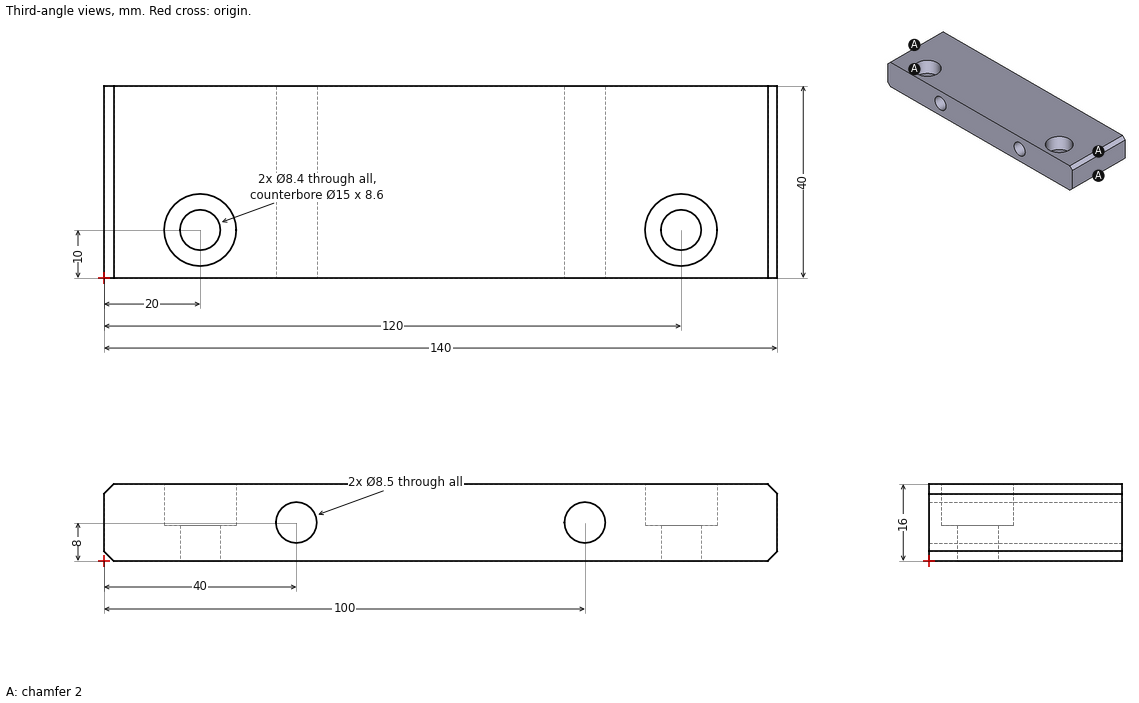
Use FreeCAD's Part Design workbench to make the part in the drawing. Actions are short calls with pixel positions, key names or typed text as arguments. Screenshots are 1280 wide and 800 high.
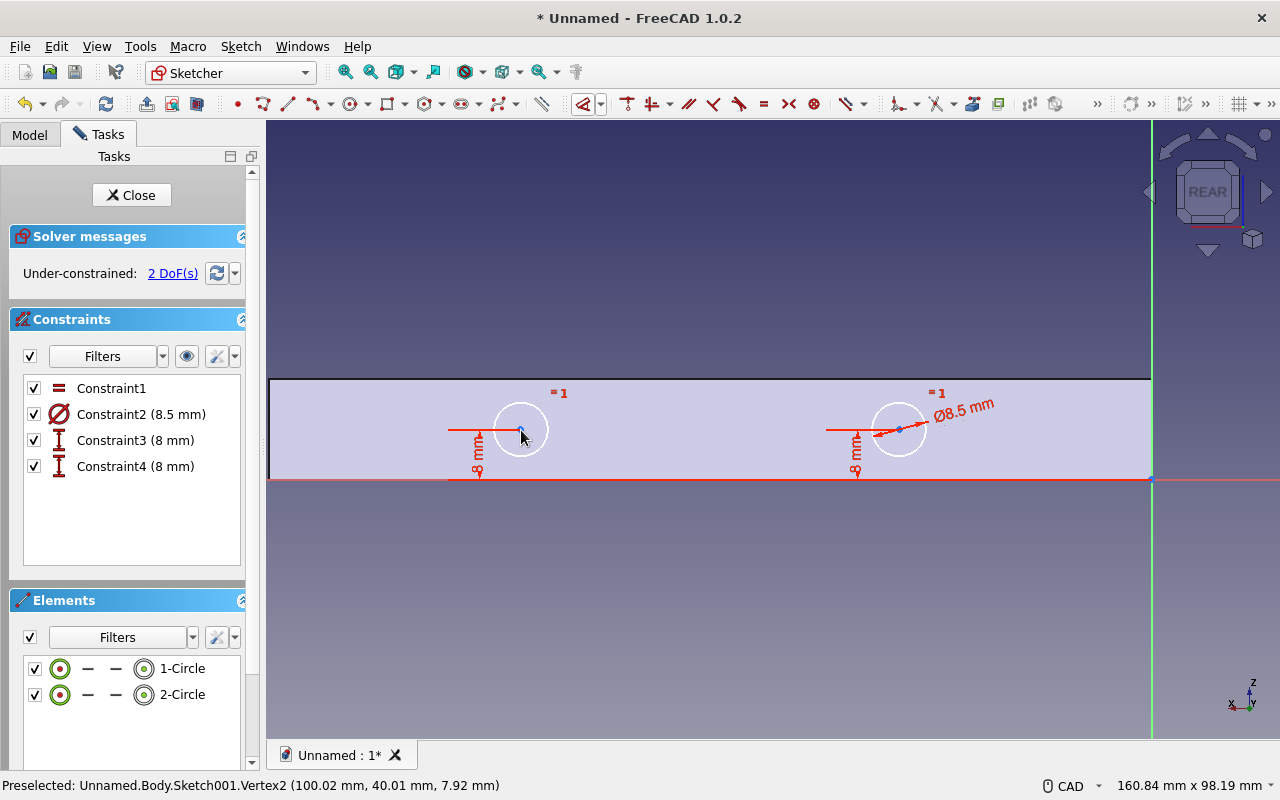
click(899, 429)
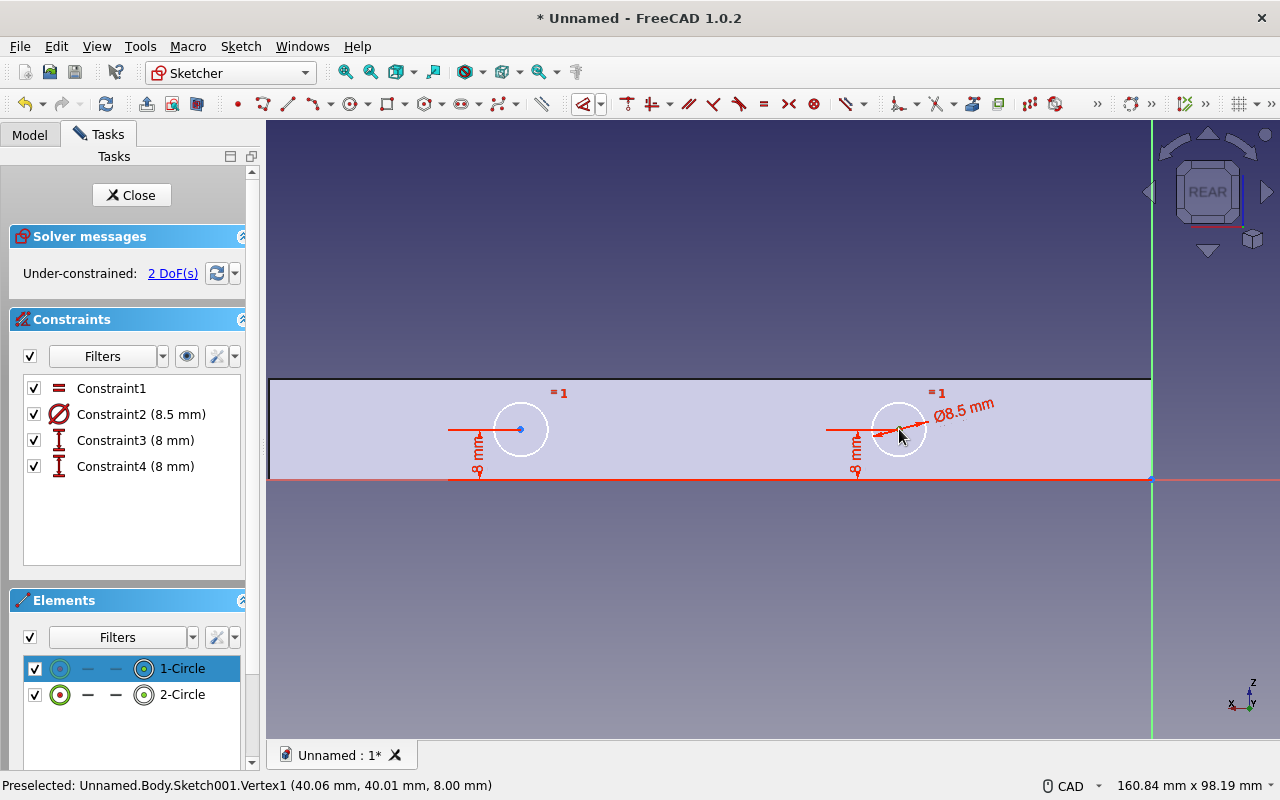
key(l)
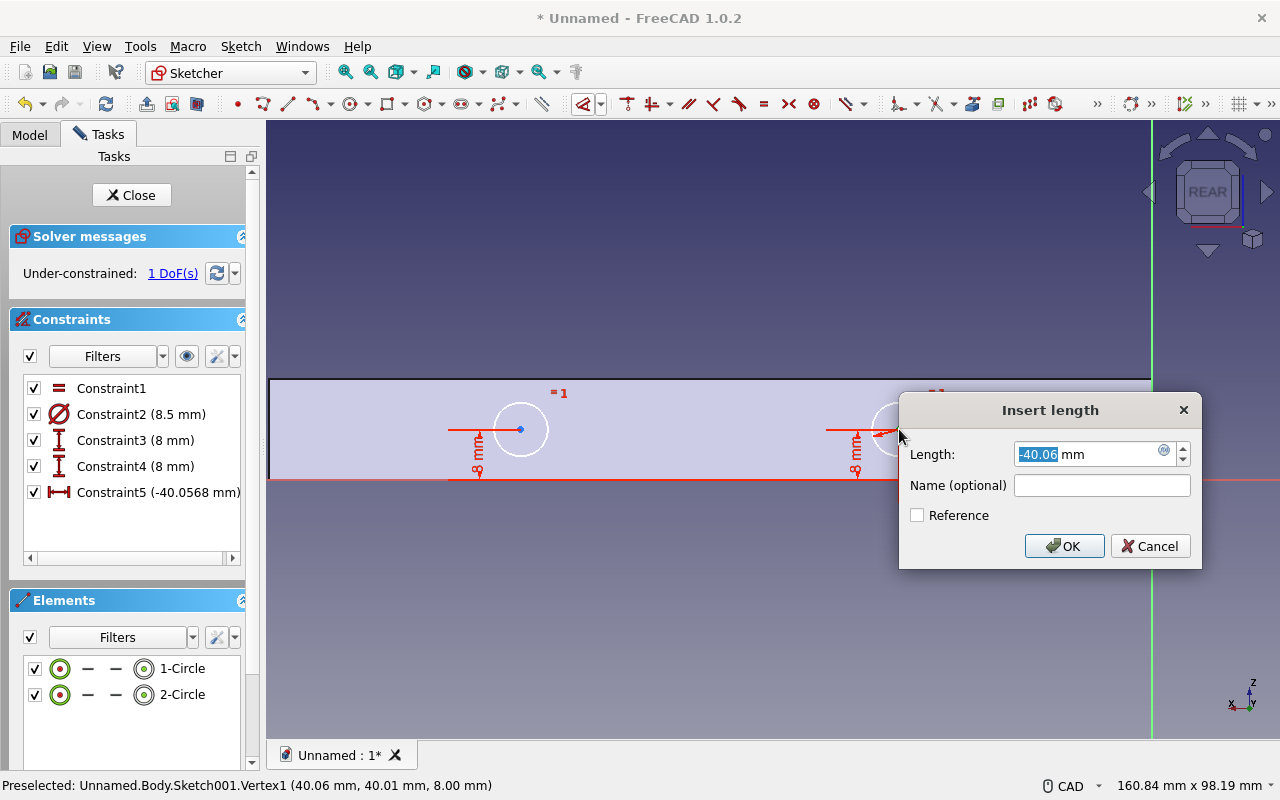
text(-40)
key(Return)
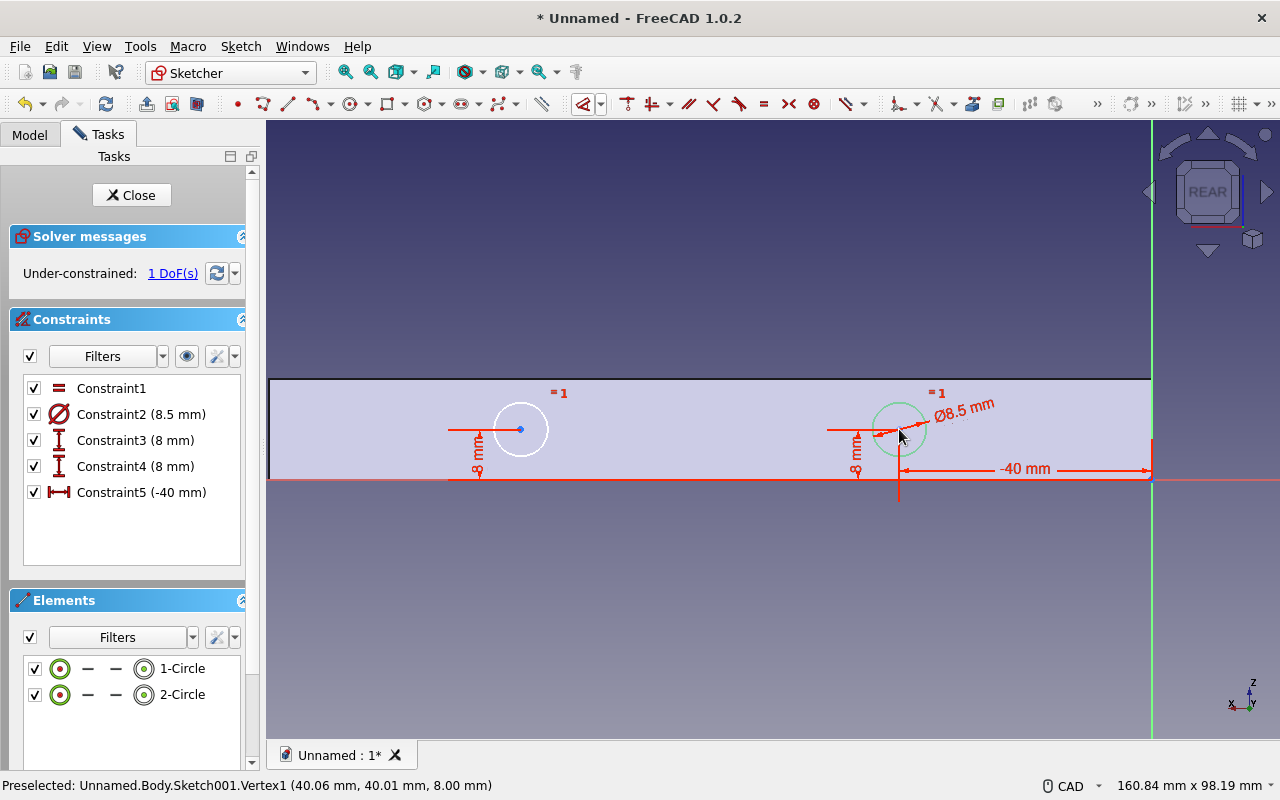
click(521, 429)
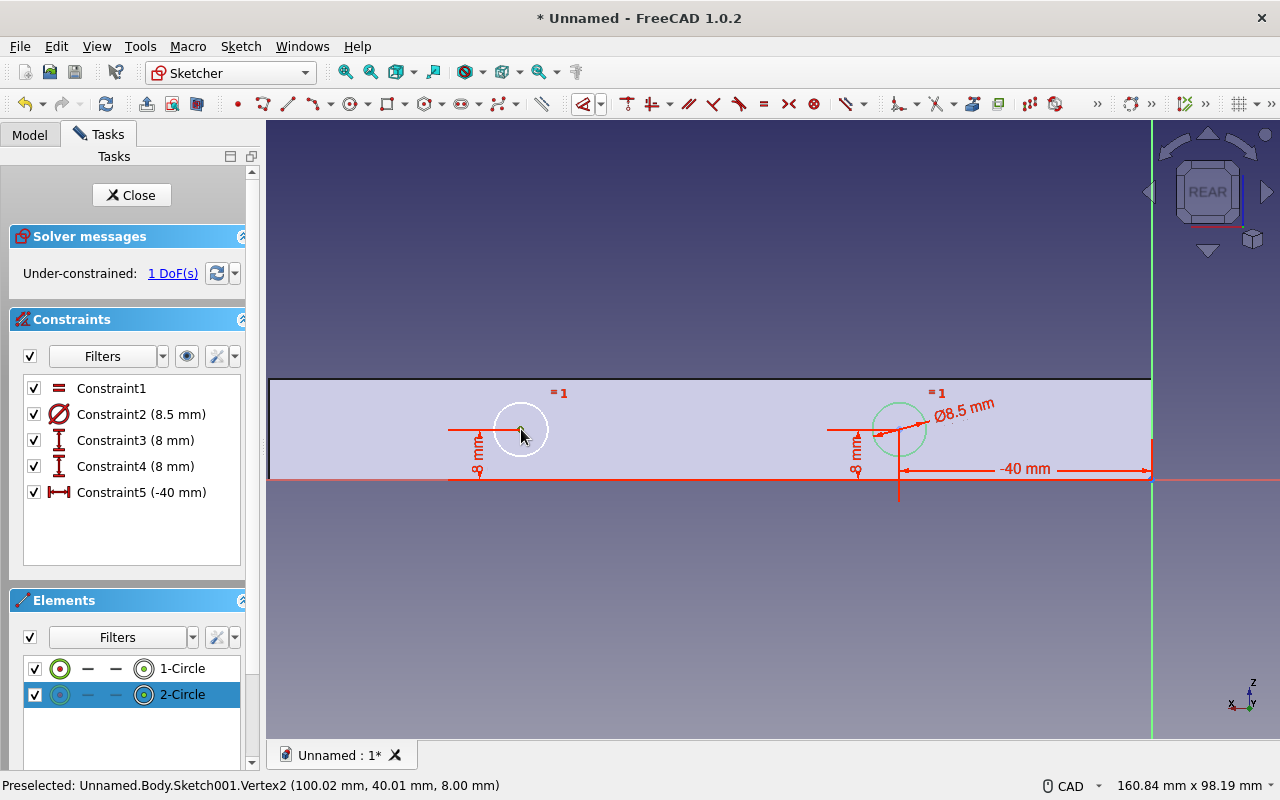
key(l)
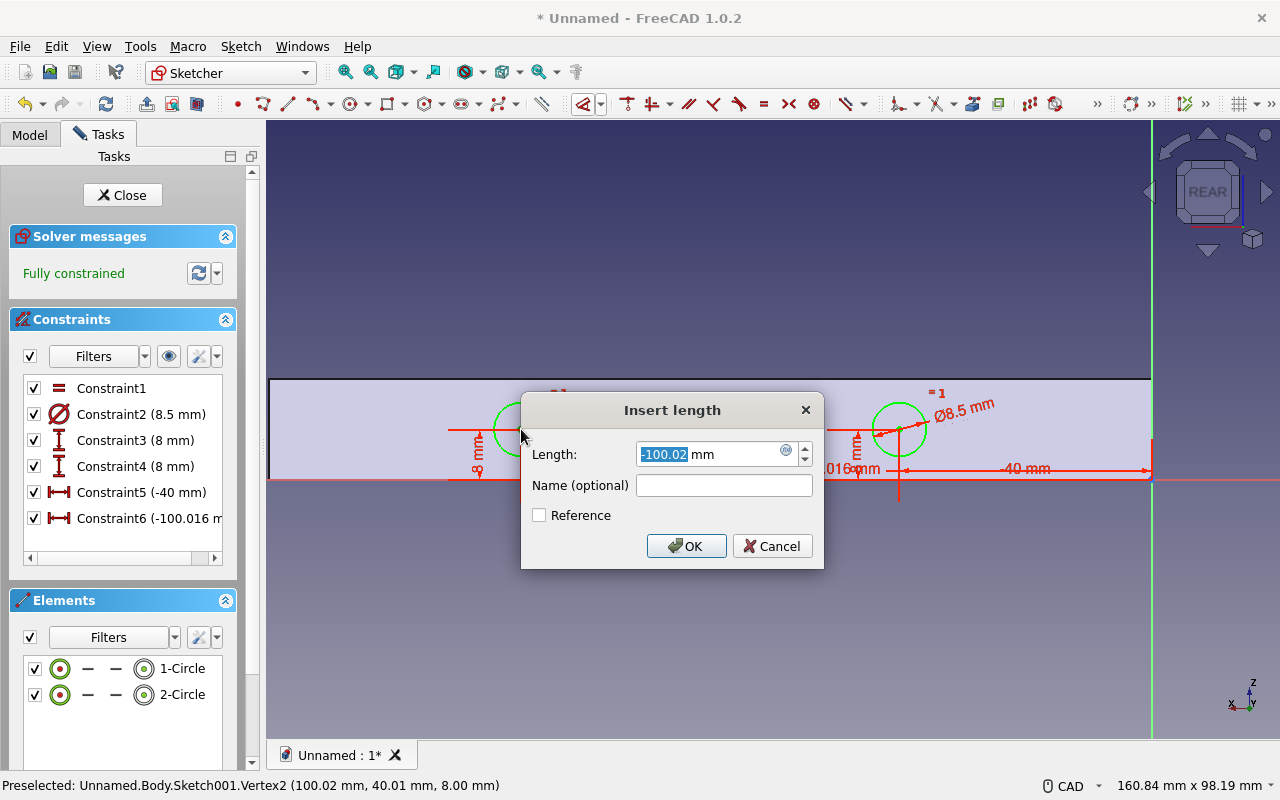
text(-100)
key(Return)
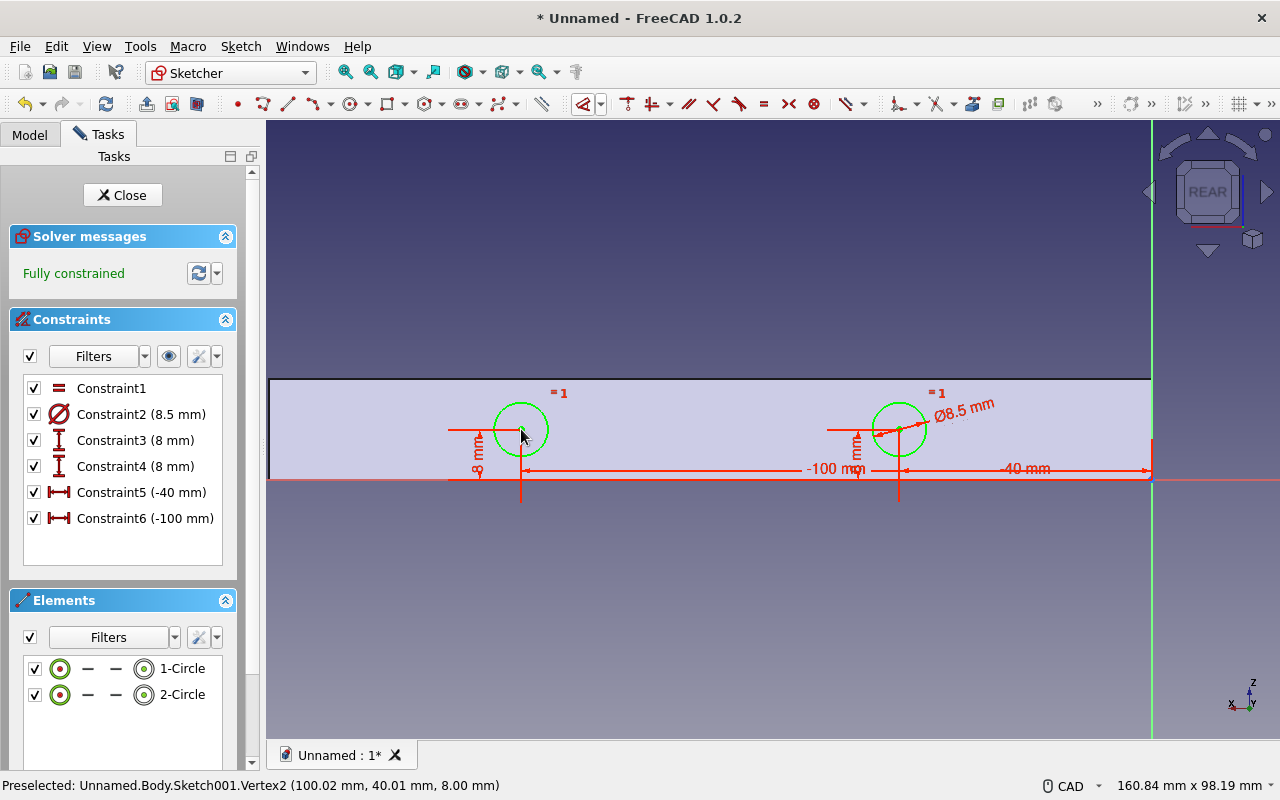
click(123, 195)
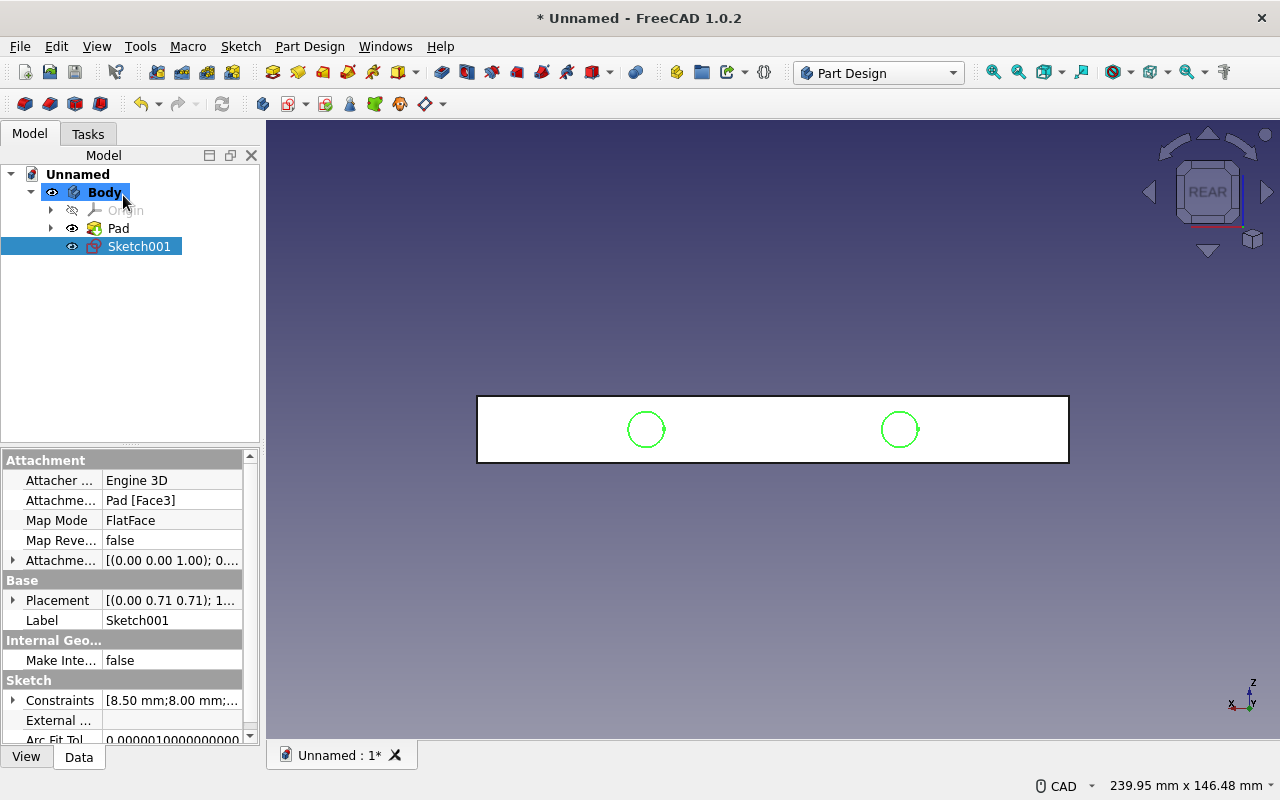
click(467, 72)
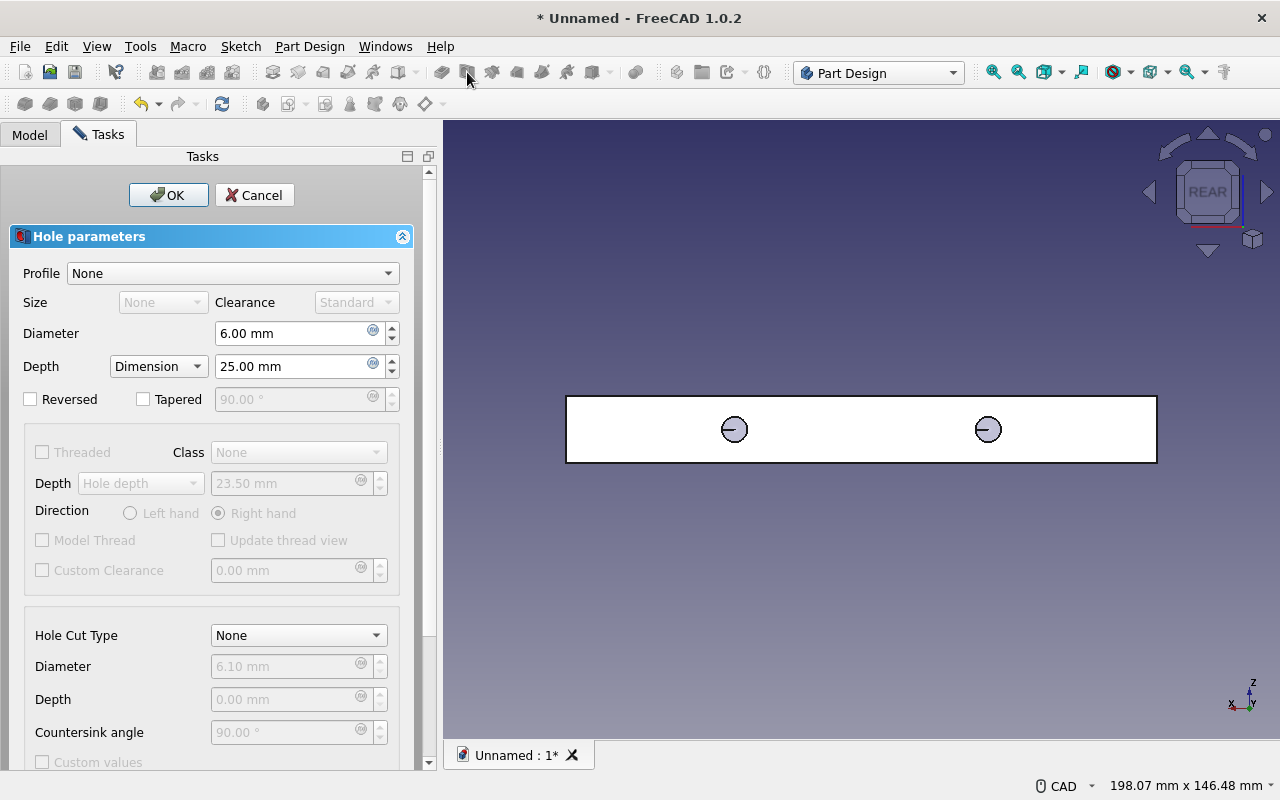
triple_click(300, 334)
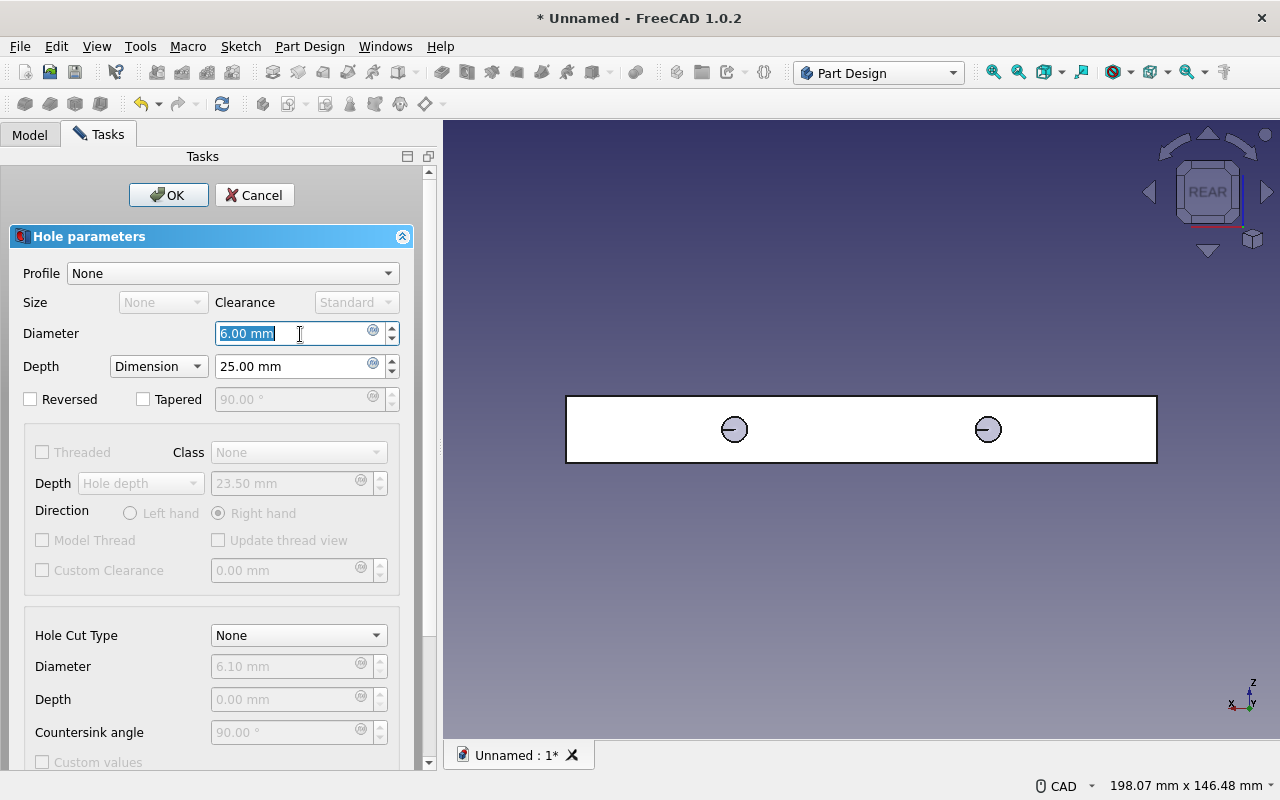
text(8.5)
key(Tab)